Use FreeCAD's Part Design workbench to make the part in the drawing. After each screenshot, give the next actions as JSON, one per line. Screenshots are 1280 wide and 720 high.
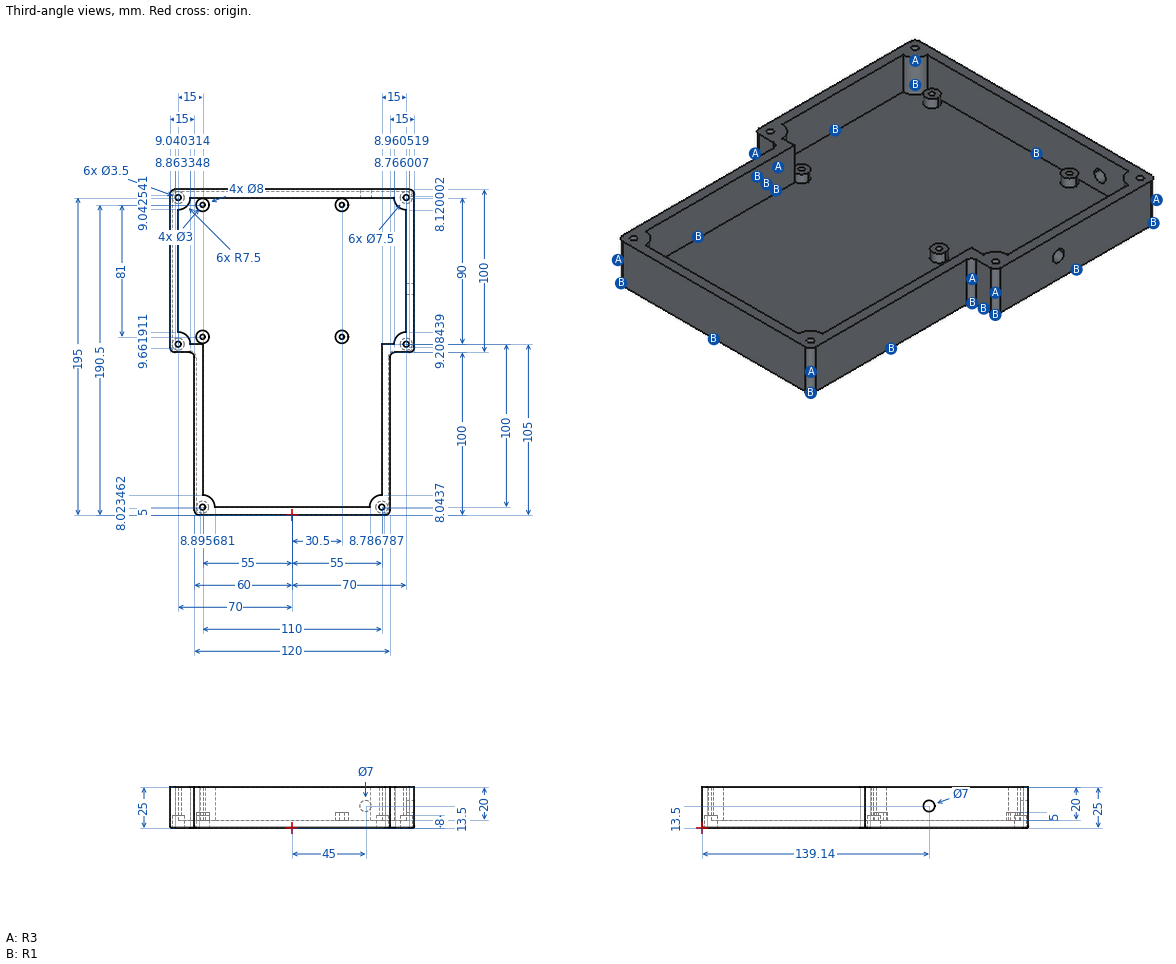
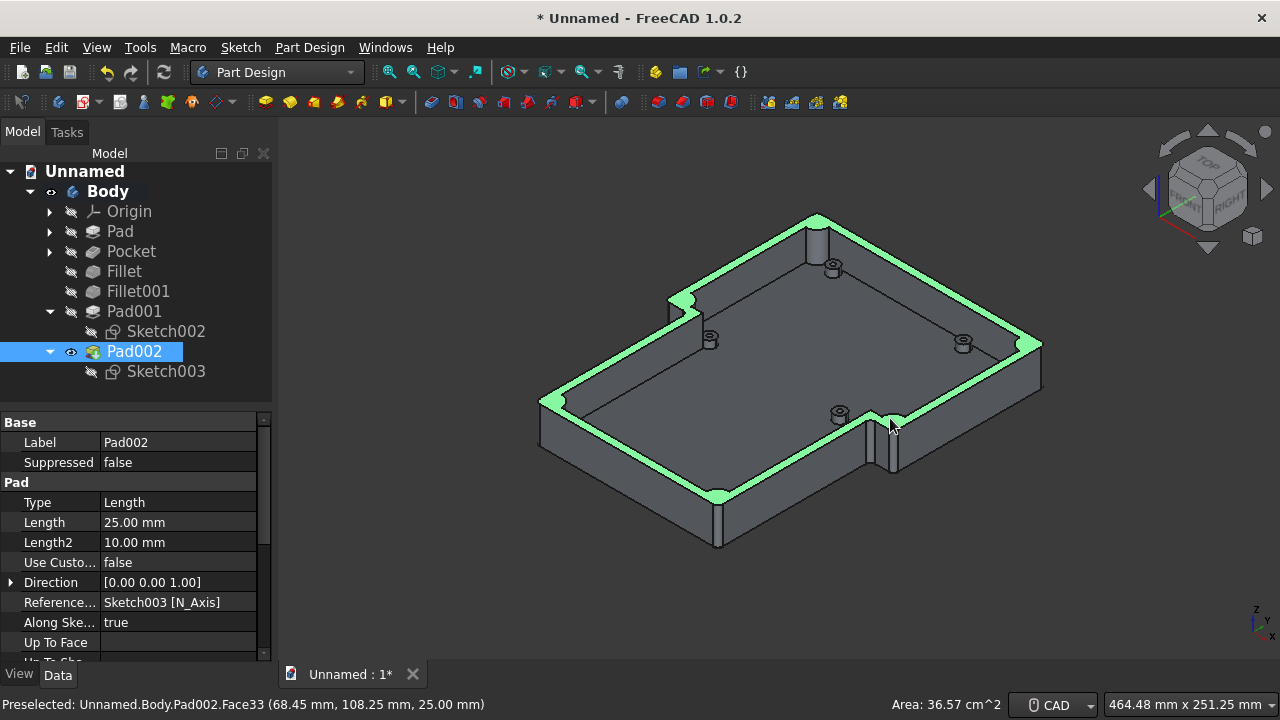
{"action": "left_click", "coordinate": [84, 102]}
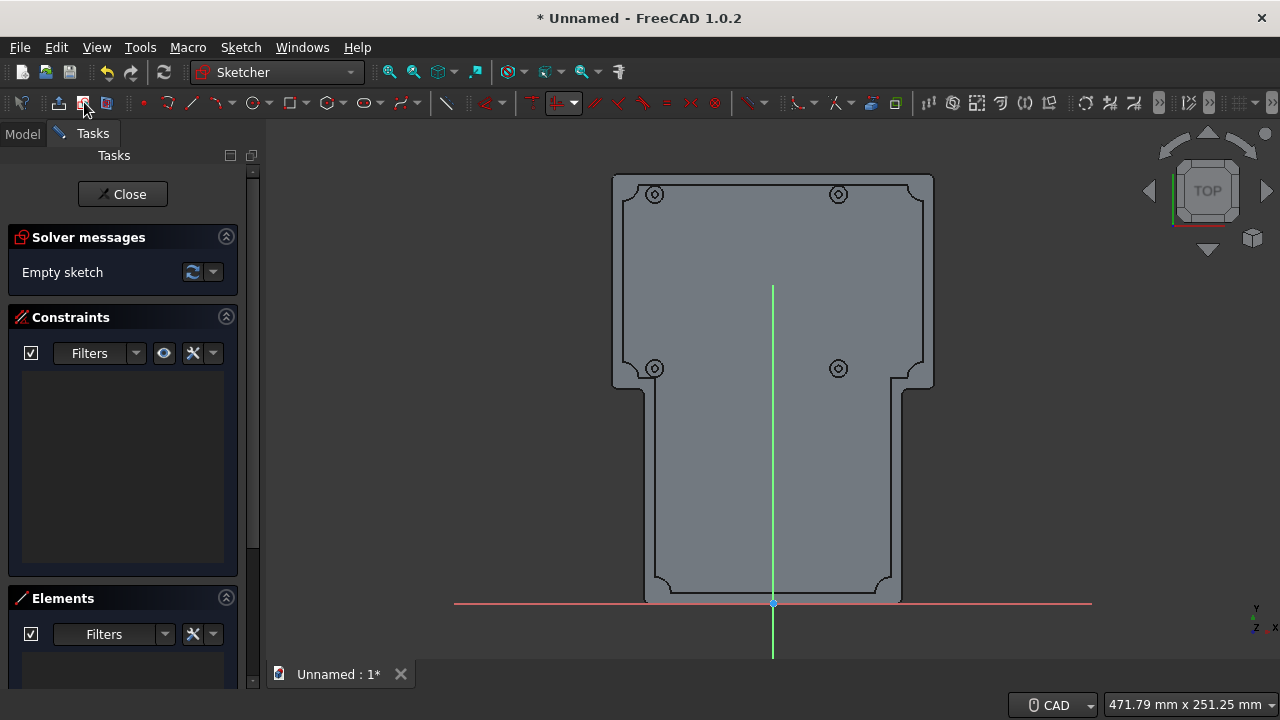
{"action": "left_click", "coordinate": [254, 104]}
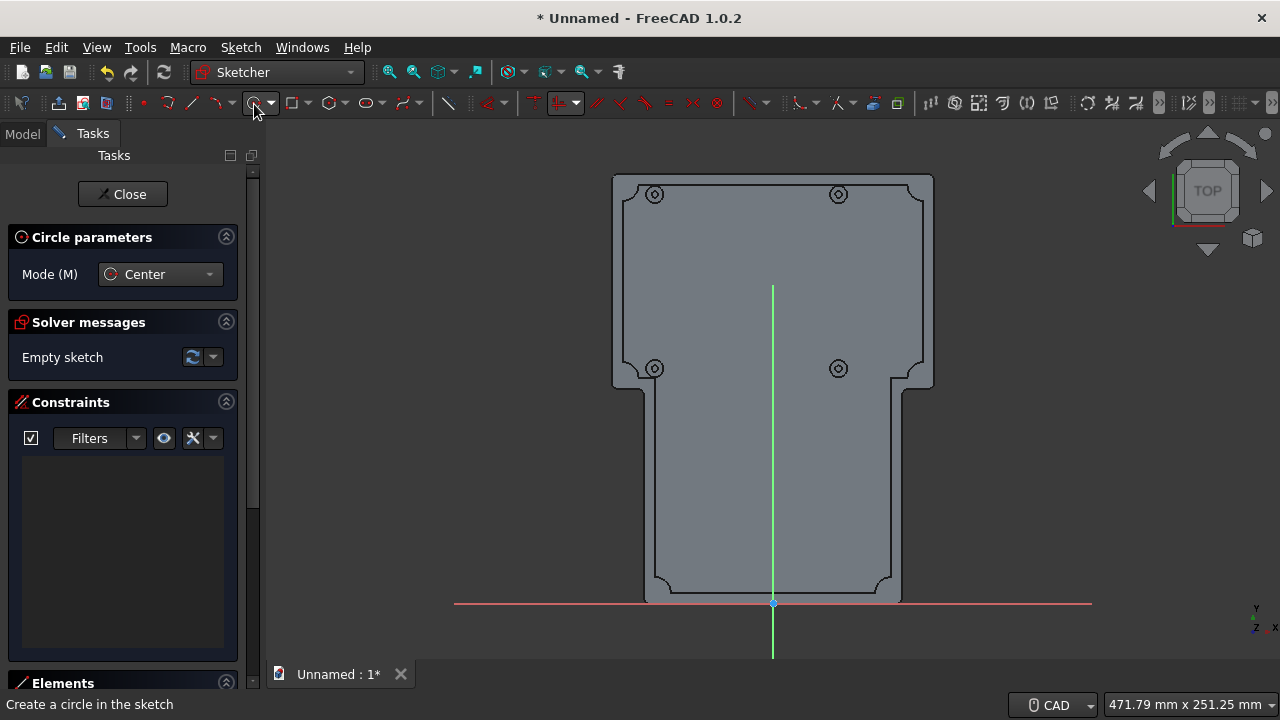
{"action": "scroll", "coordinate": [623, 185], "scroll_direction": "up", "scroll_amount": 9}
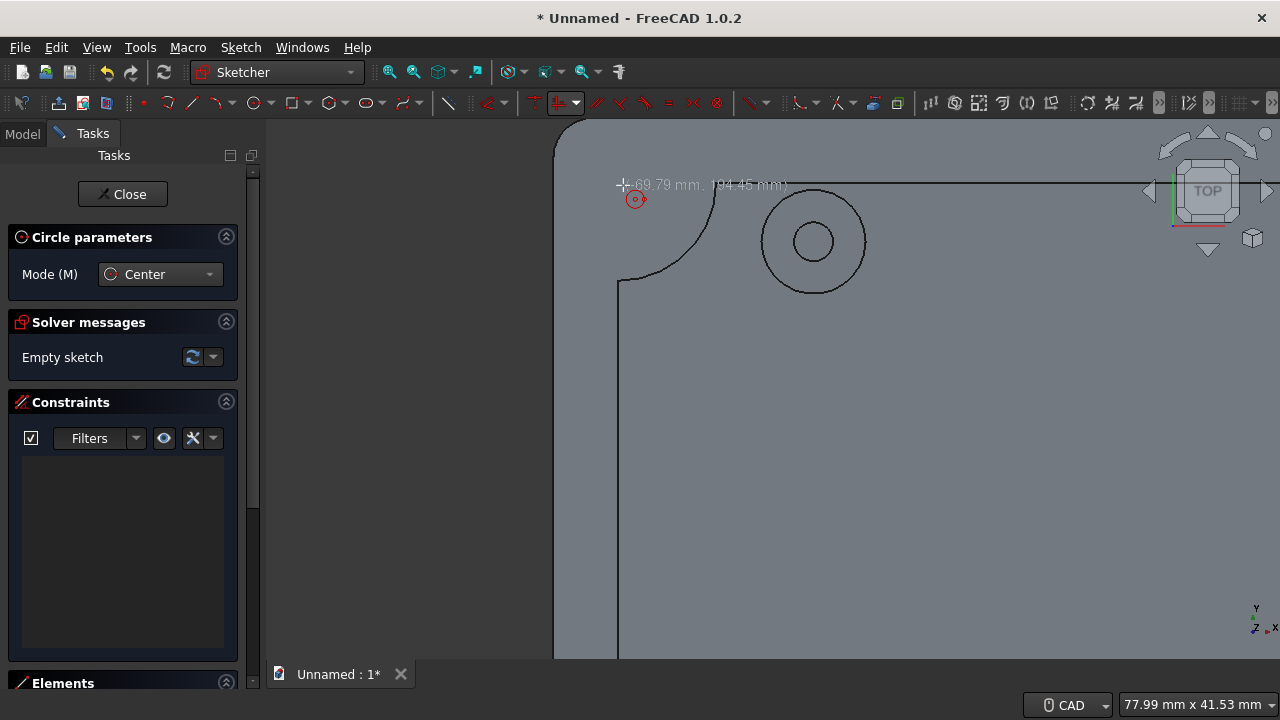
{"action": "scroll", "coordinate": [576, 225], "scroll_direction": "down", "scroll_amount": 10}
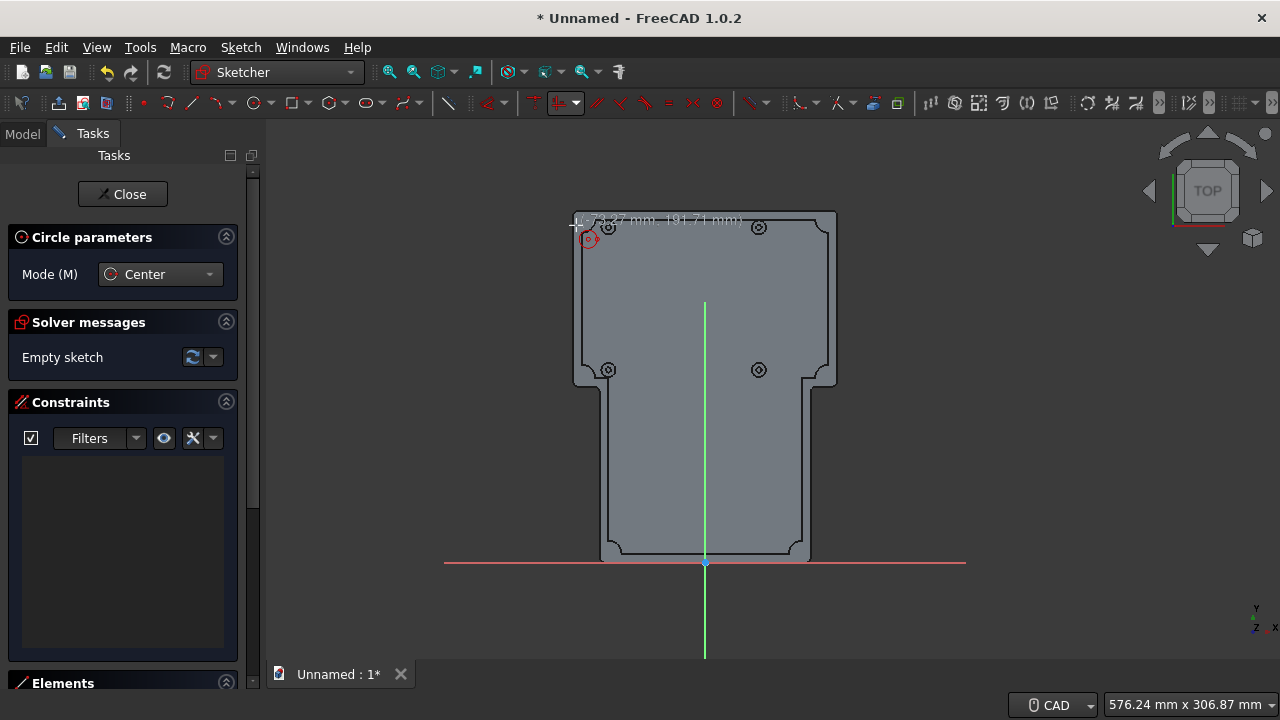
{"action": "left_click", "coordinate": [582, 220]}
{"action": "mouse_move", "coordinate": [584, 217]}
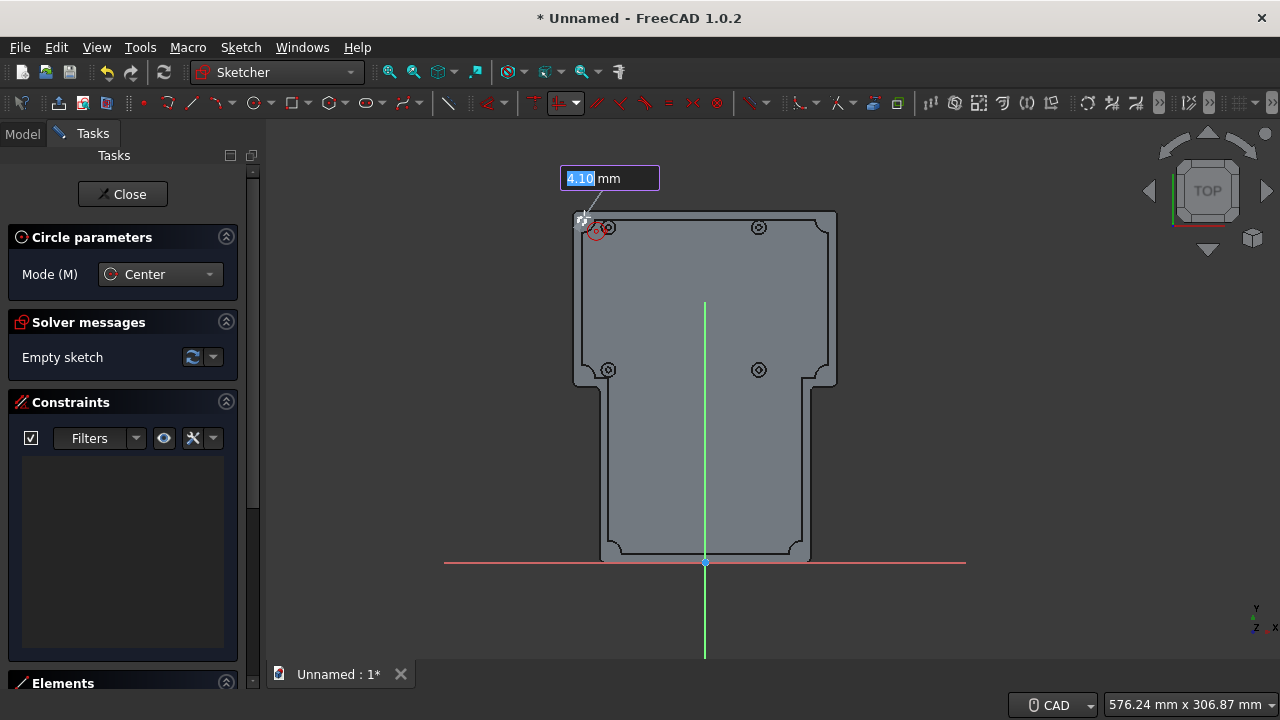
{"action": "type", "text": "3.5"}
{"action": "key", "text": "Return"}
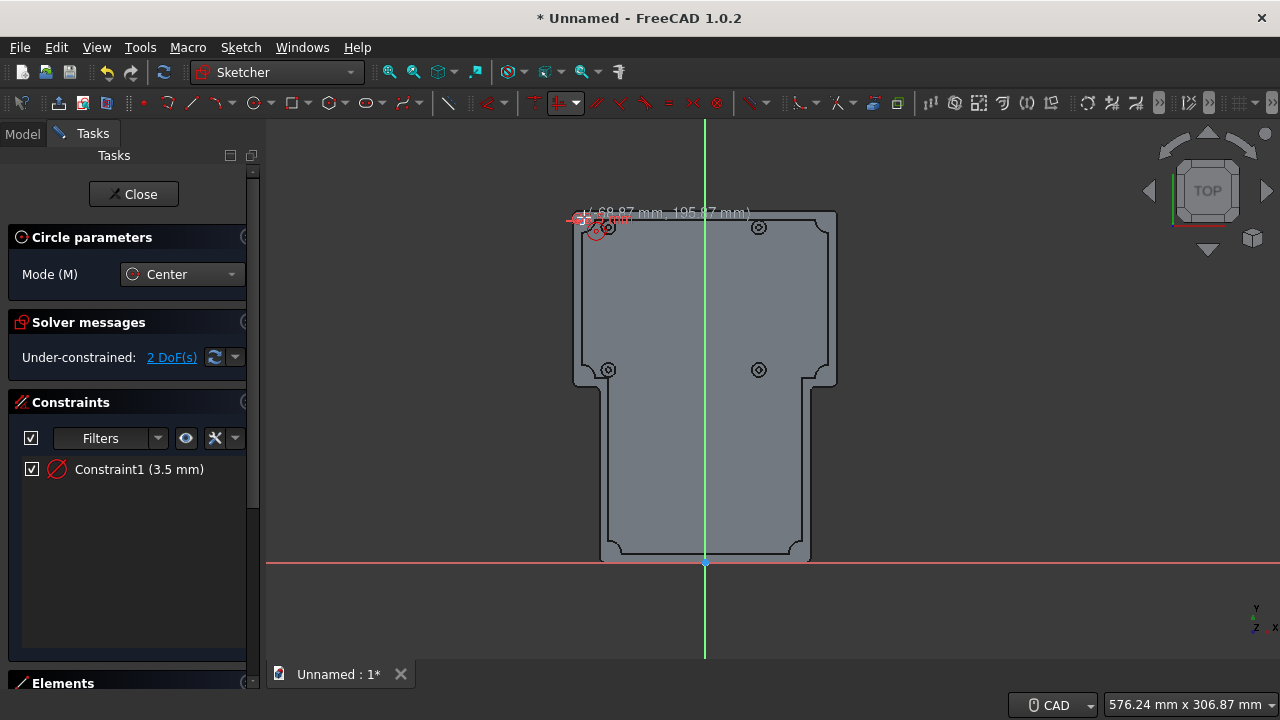
{"action": "scroll", "coordinate": [582, 378], "scroll_direction": "up", "scroll_amount": 10}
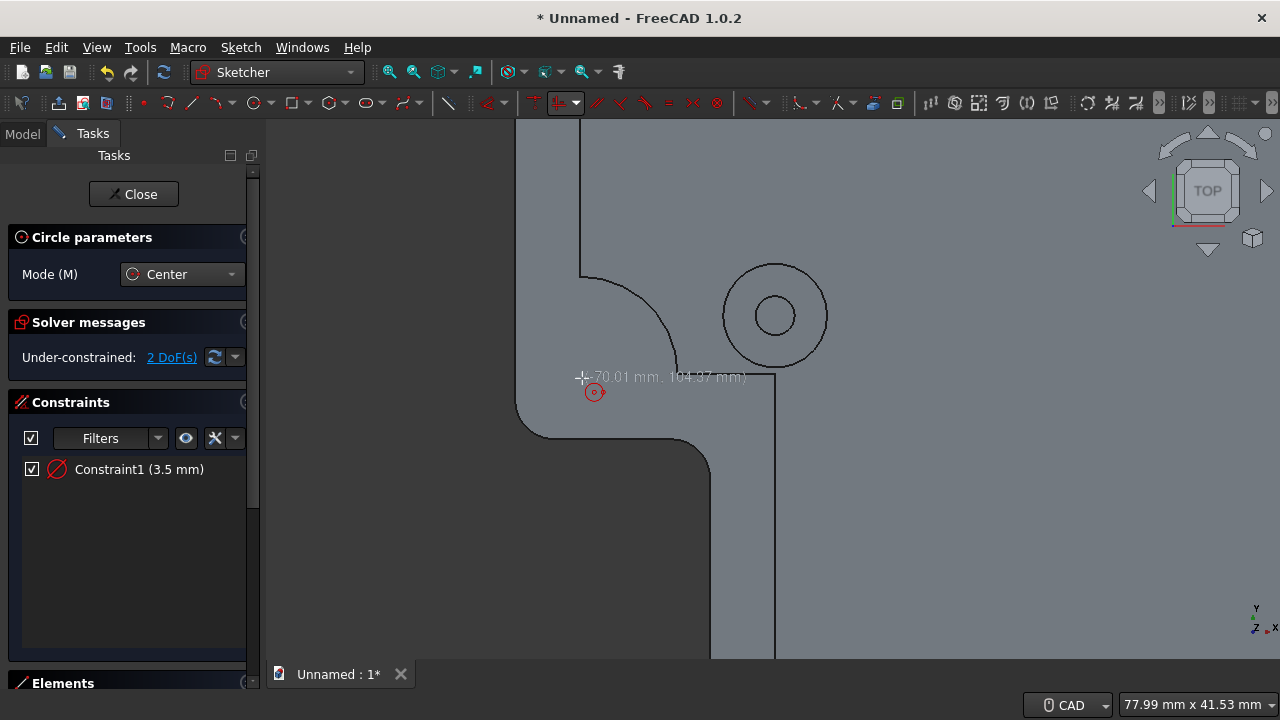
{"action": "scroll", "coordinate": [582, 378], "scroll_direction": "down", "scroll_amount": 10}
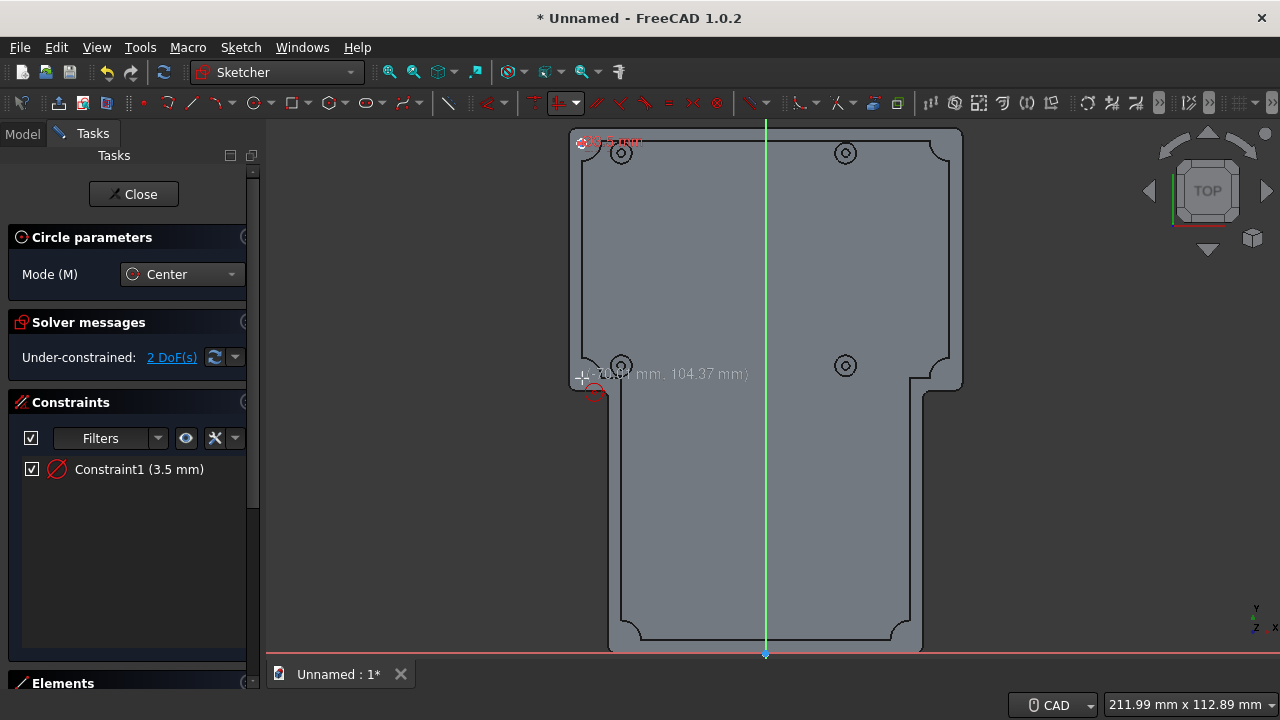
{"action": "left_click", "coordinate": [582, 378]}
{"action": "mouse_move", "coordinate": [584, 376]}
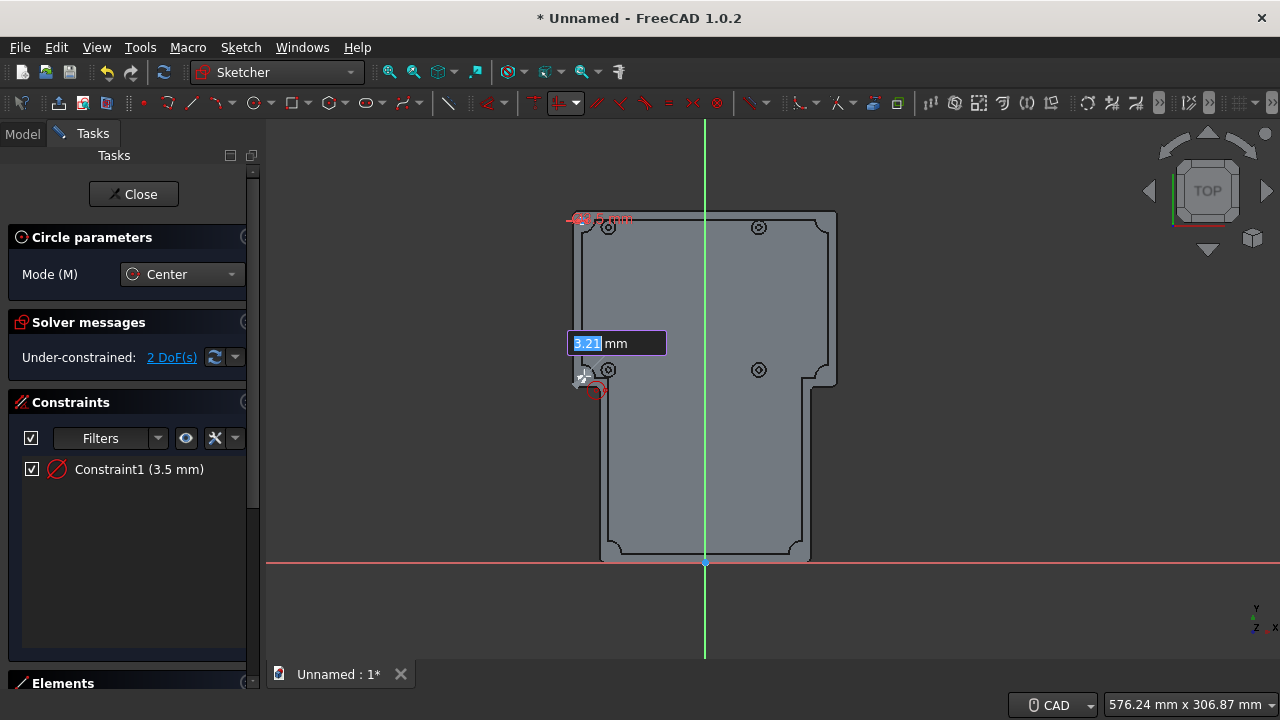
{"action": "type", "text": "3.5"}
{"action": "key", "text": "Return"}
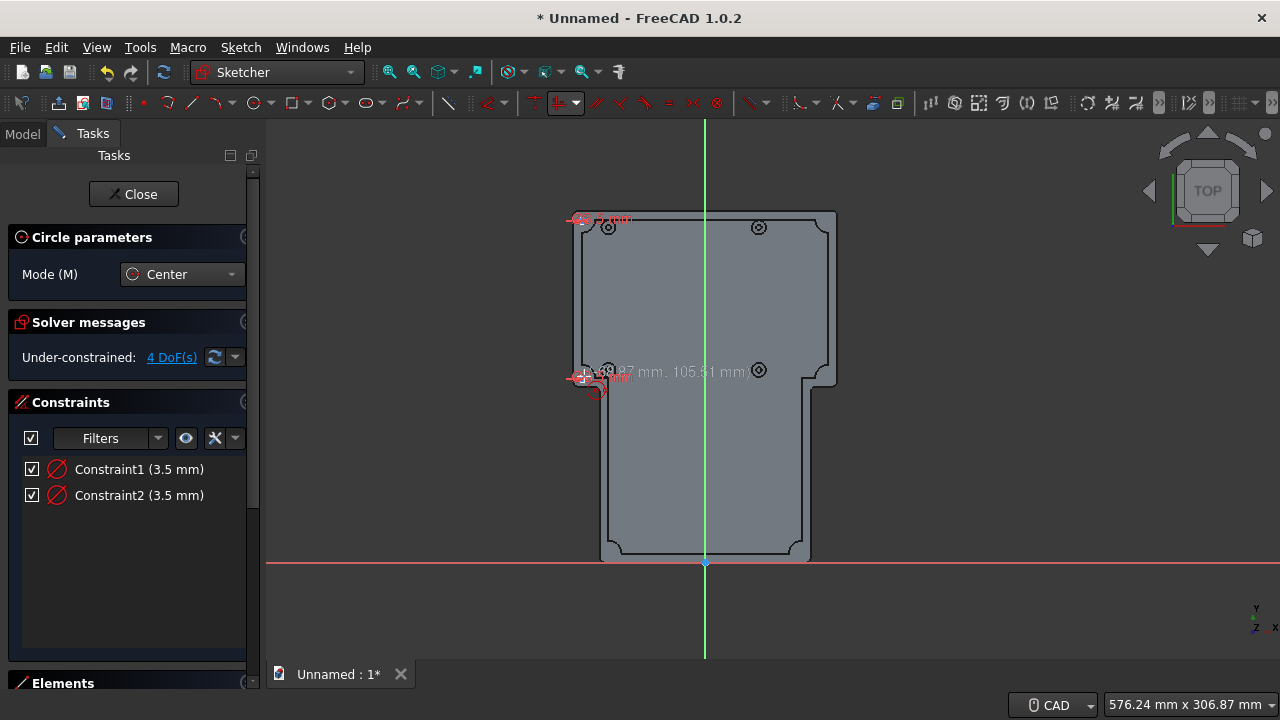
{"action": "scroll", "coordinate": [608, 554], "scroll_direction": "up", "scroll_amount": 10}